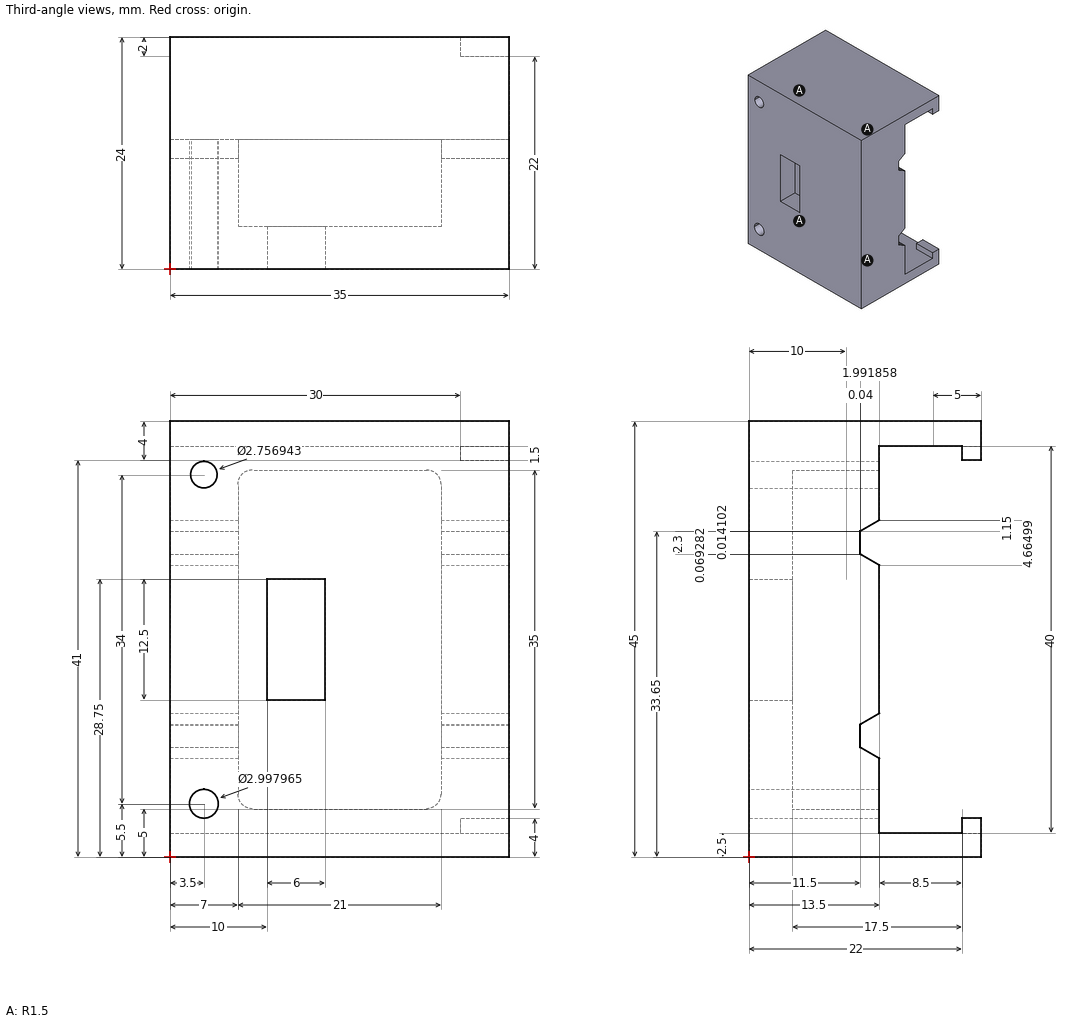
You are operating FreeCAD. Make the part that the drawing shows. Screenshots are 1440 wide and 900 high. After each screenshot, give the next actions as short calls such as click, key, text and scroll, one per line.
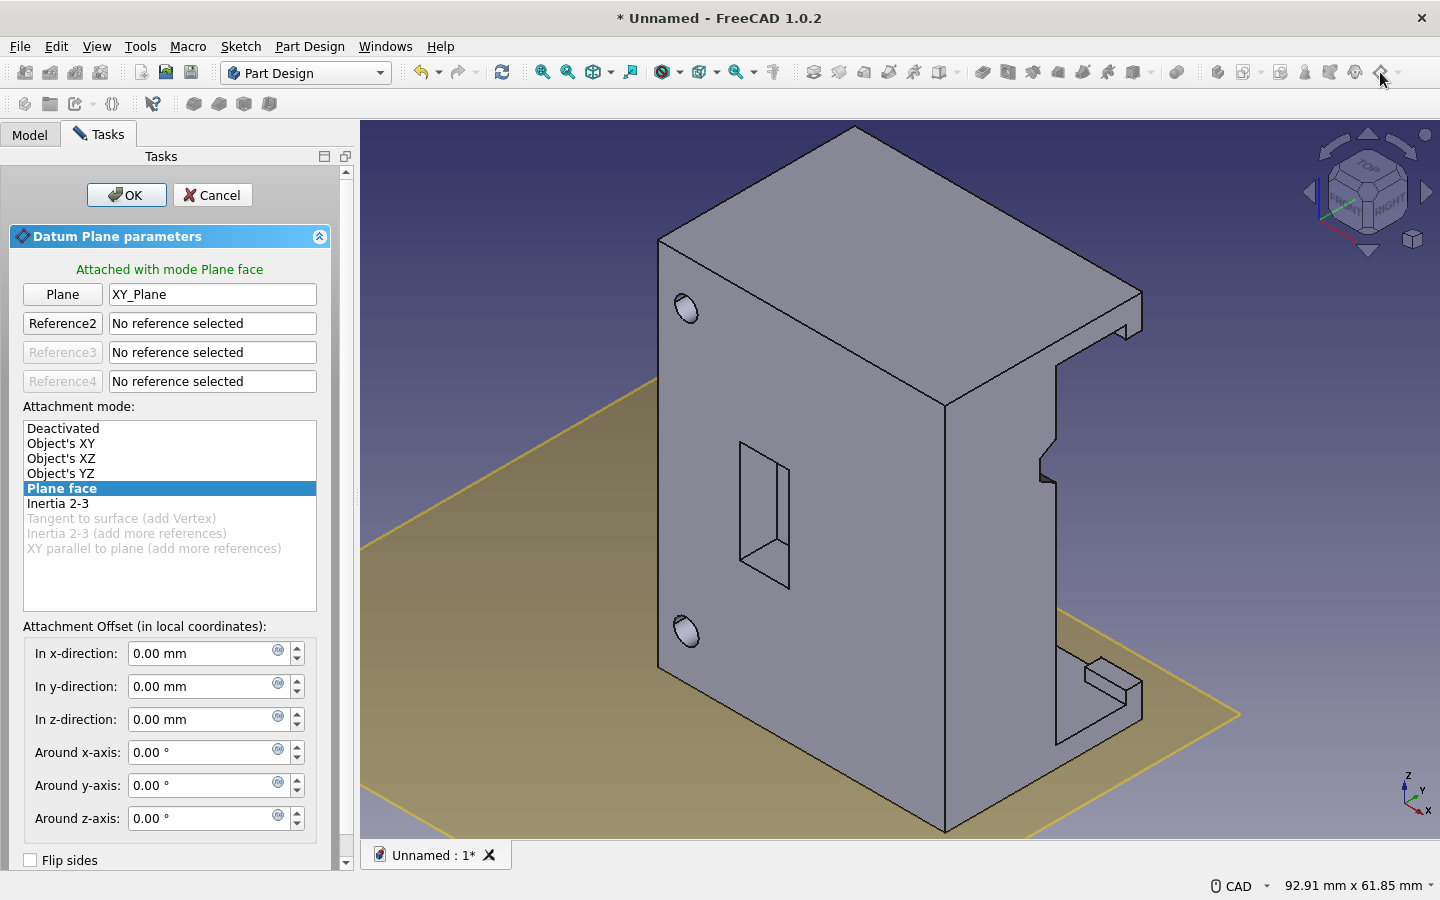
triple_click(210, 720)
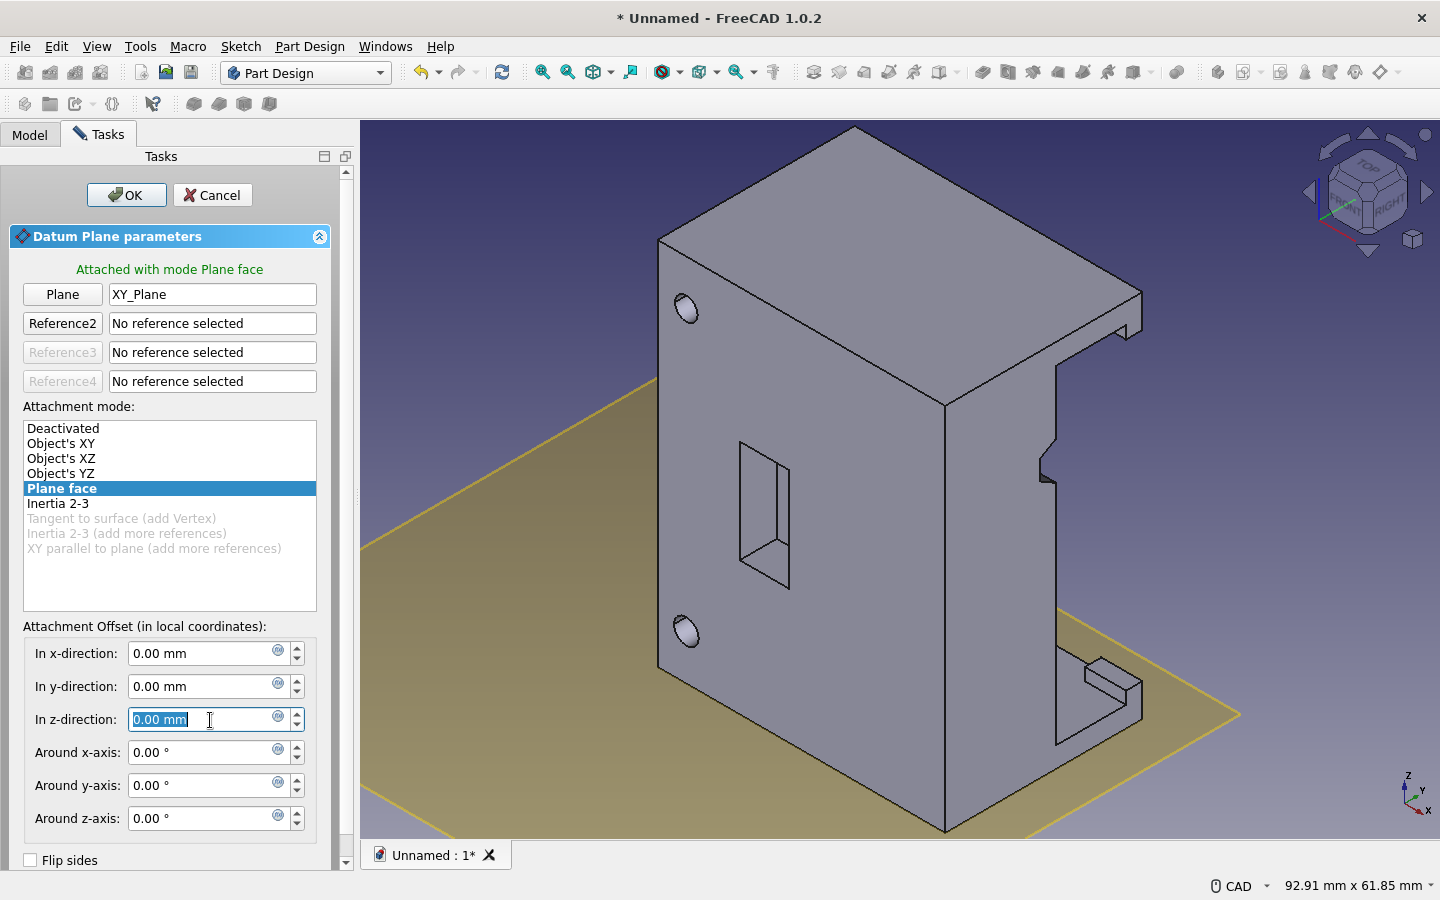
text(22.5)
key(Tab)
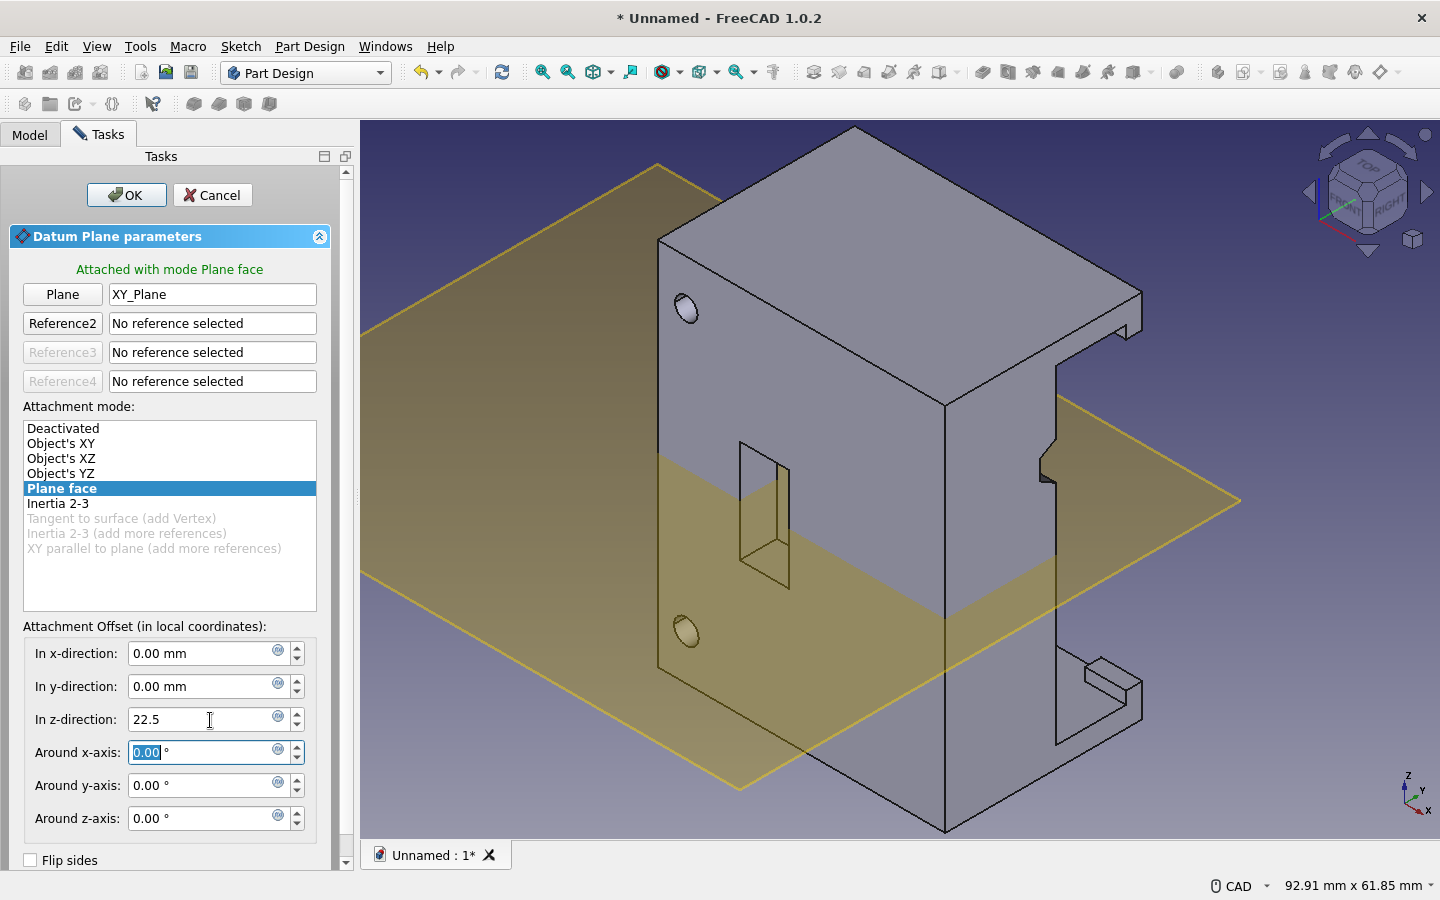
click(127, 195)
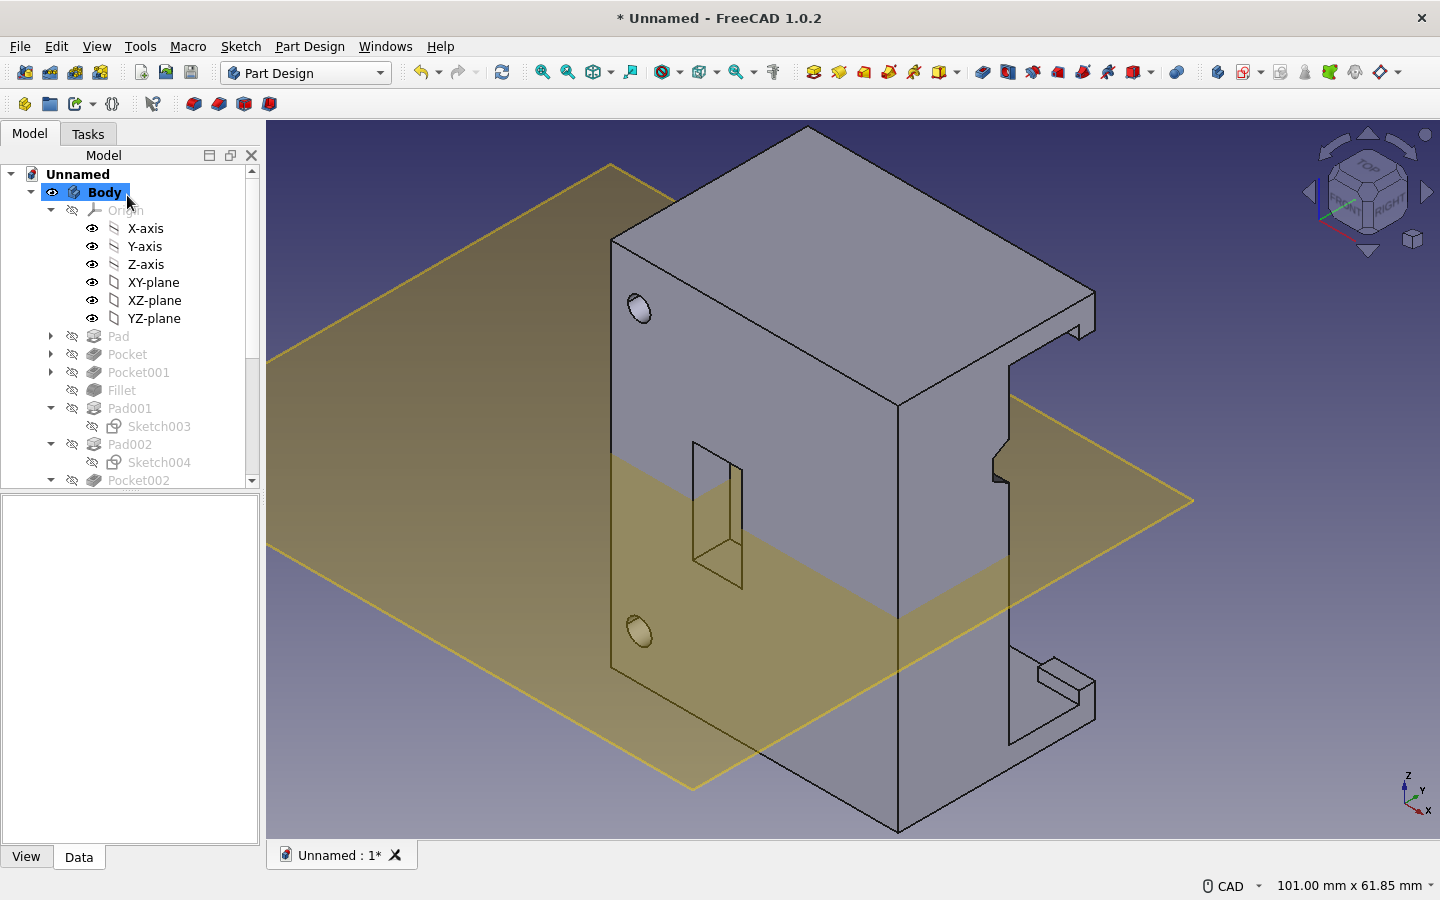
scroll(101, 332, down, 3)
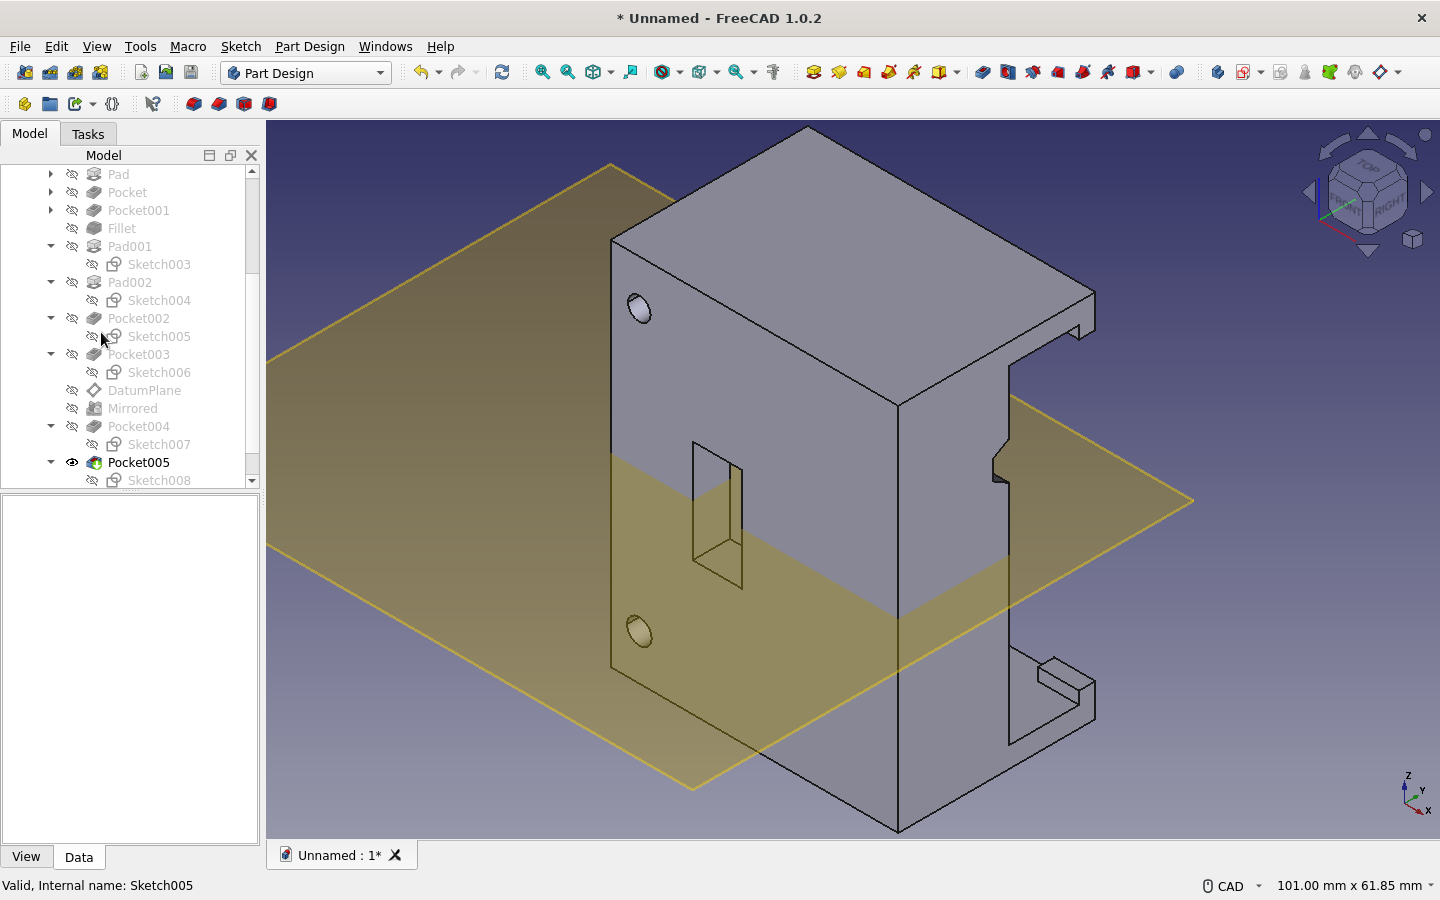
click(117, 462)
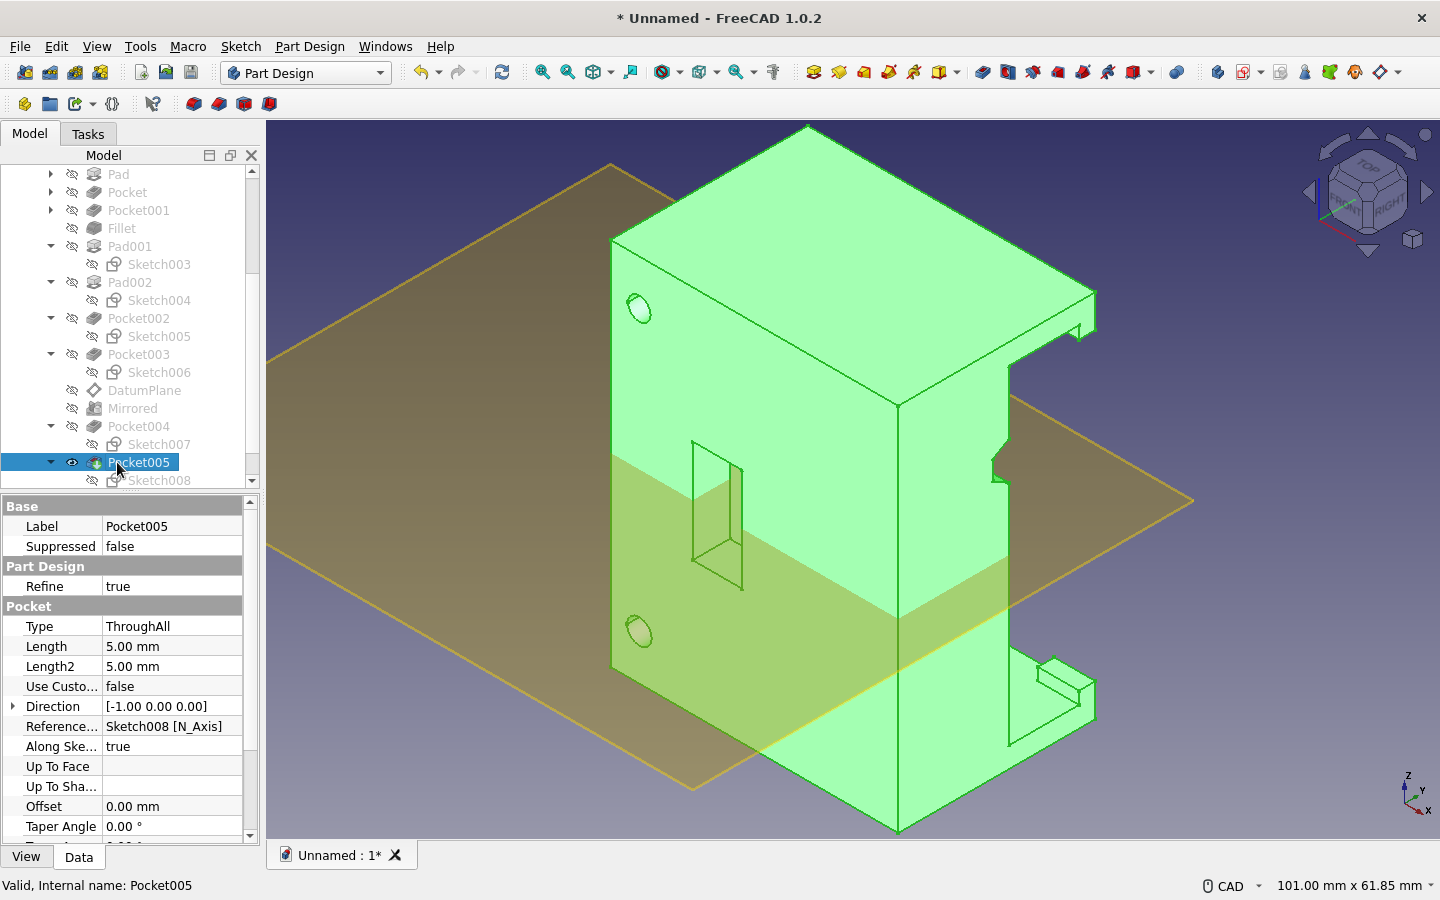
click(25, 72)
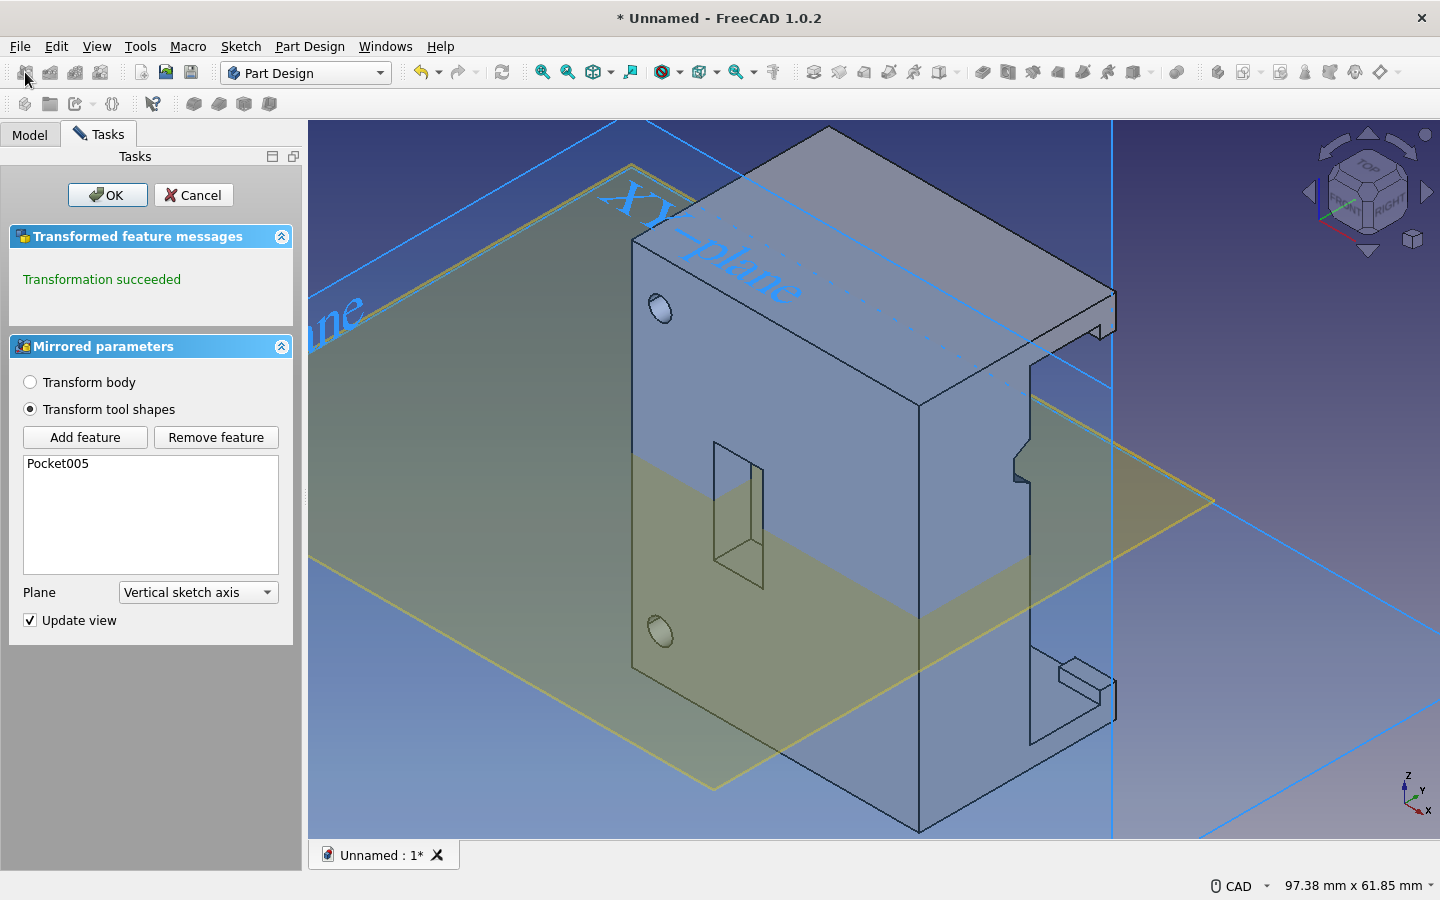
click(199, 592)